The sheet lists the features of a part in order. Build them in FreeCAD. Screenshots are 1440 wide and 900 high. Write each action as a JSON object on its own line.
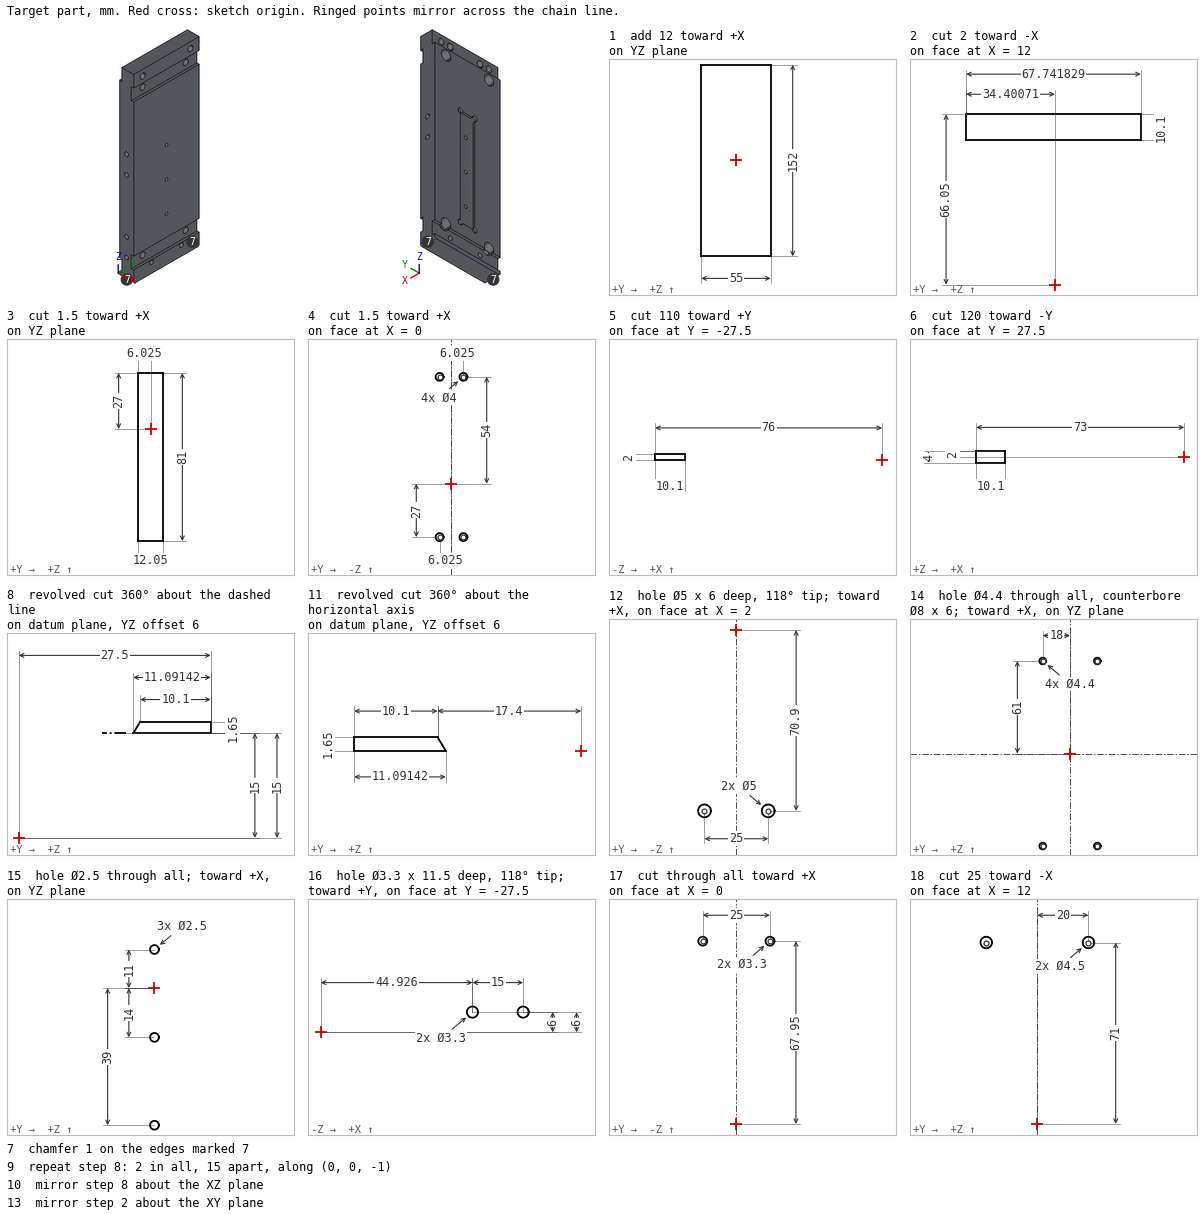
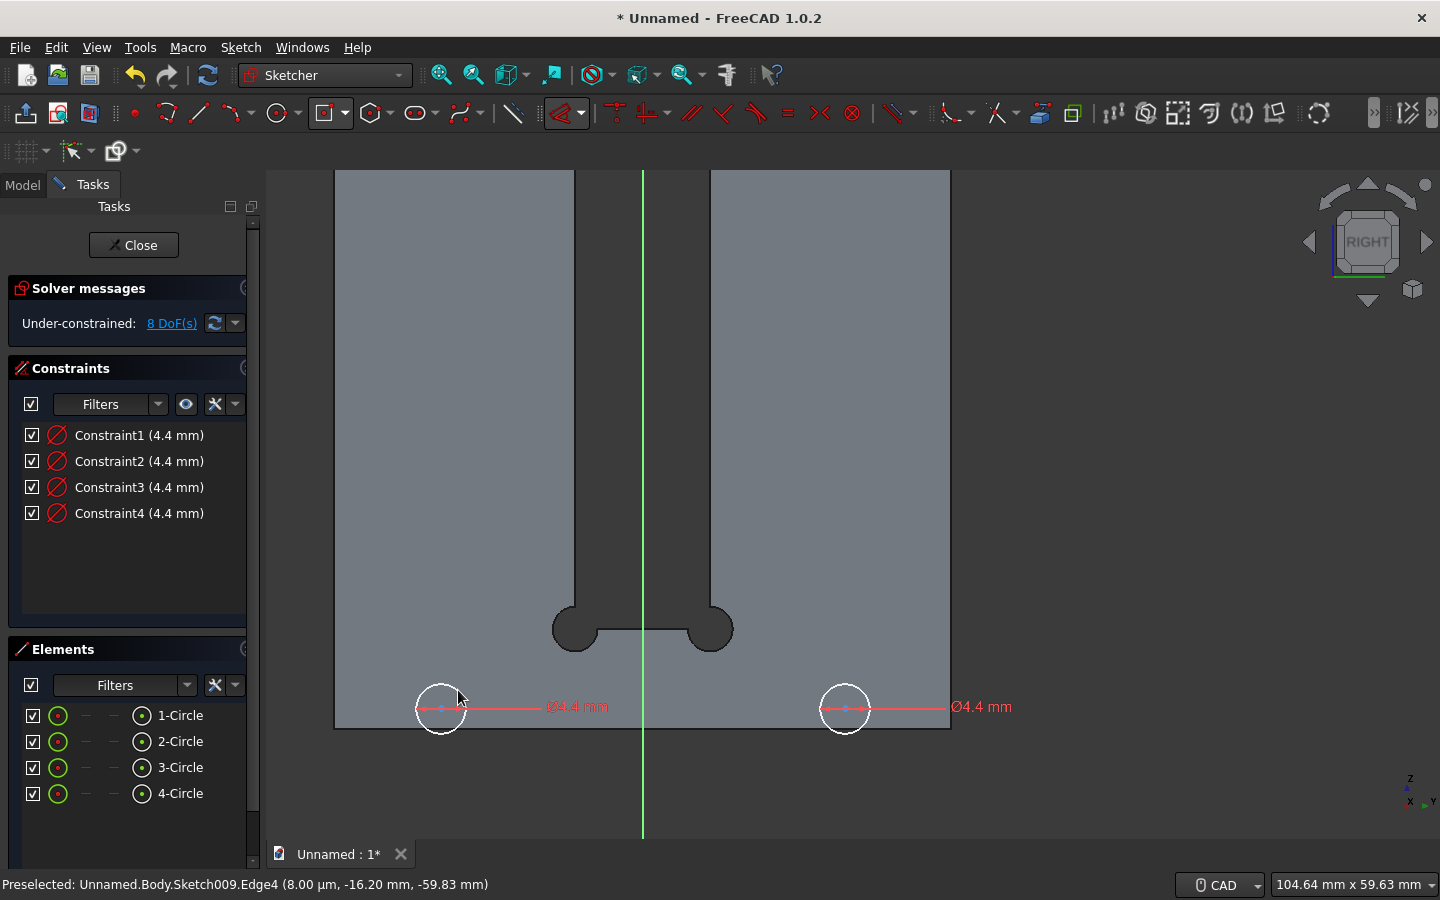
{"action": "scroll", "coordinate": [846, 712], "scroll_direction": "down", "scroll_amount": 6}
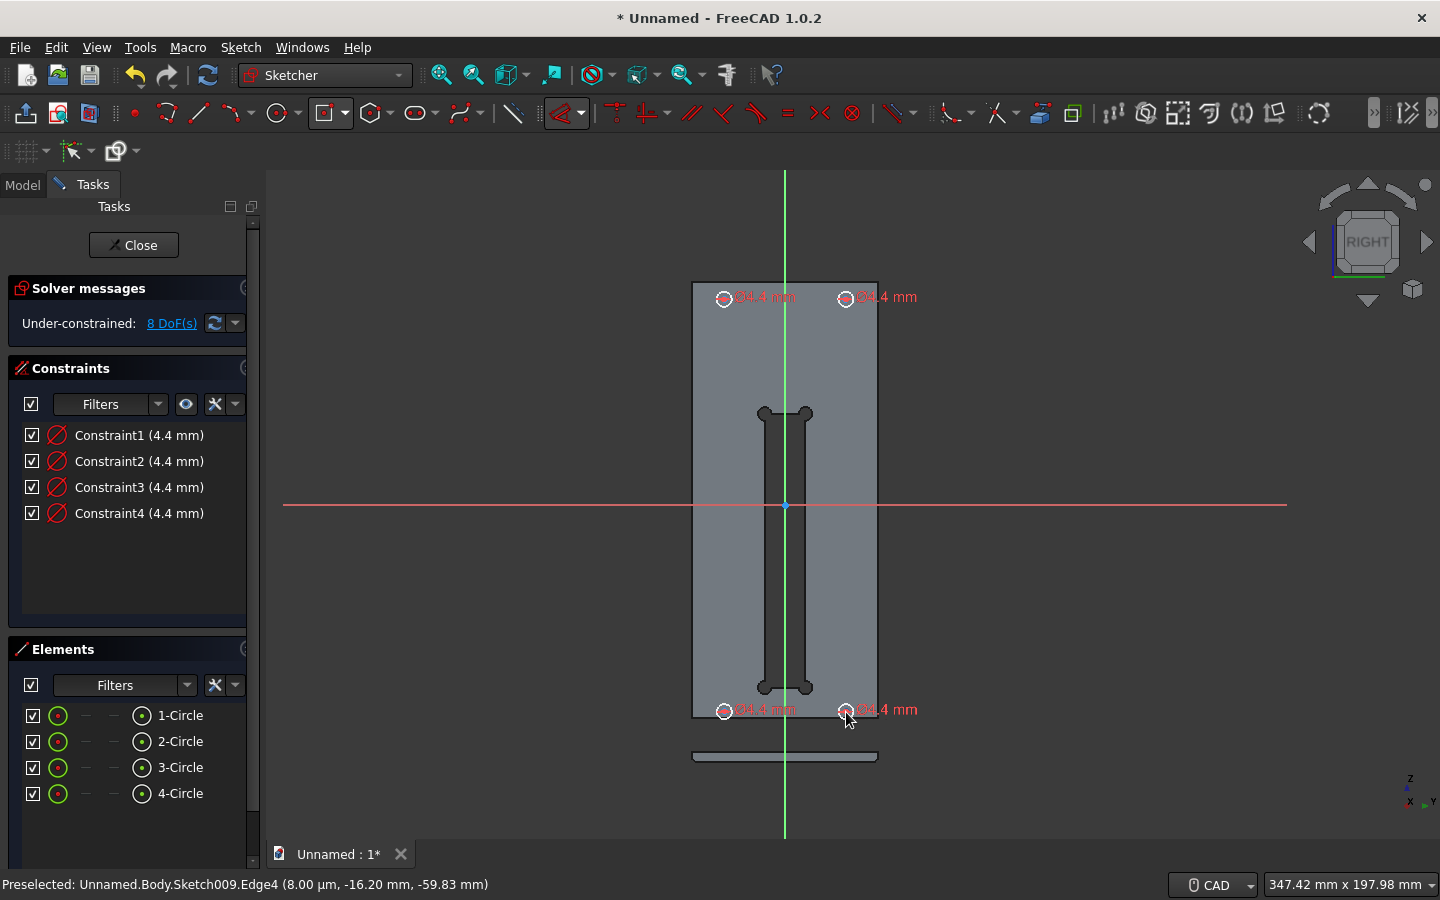
{"action": "left_click", "coordinate": [724, 299]}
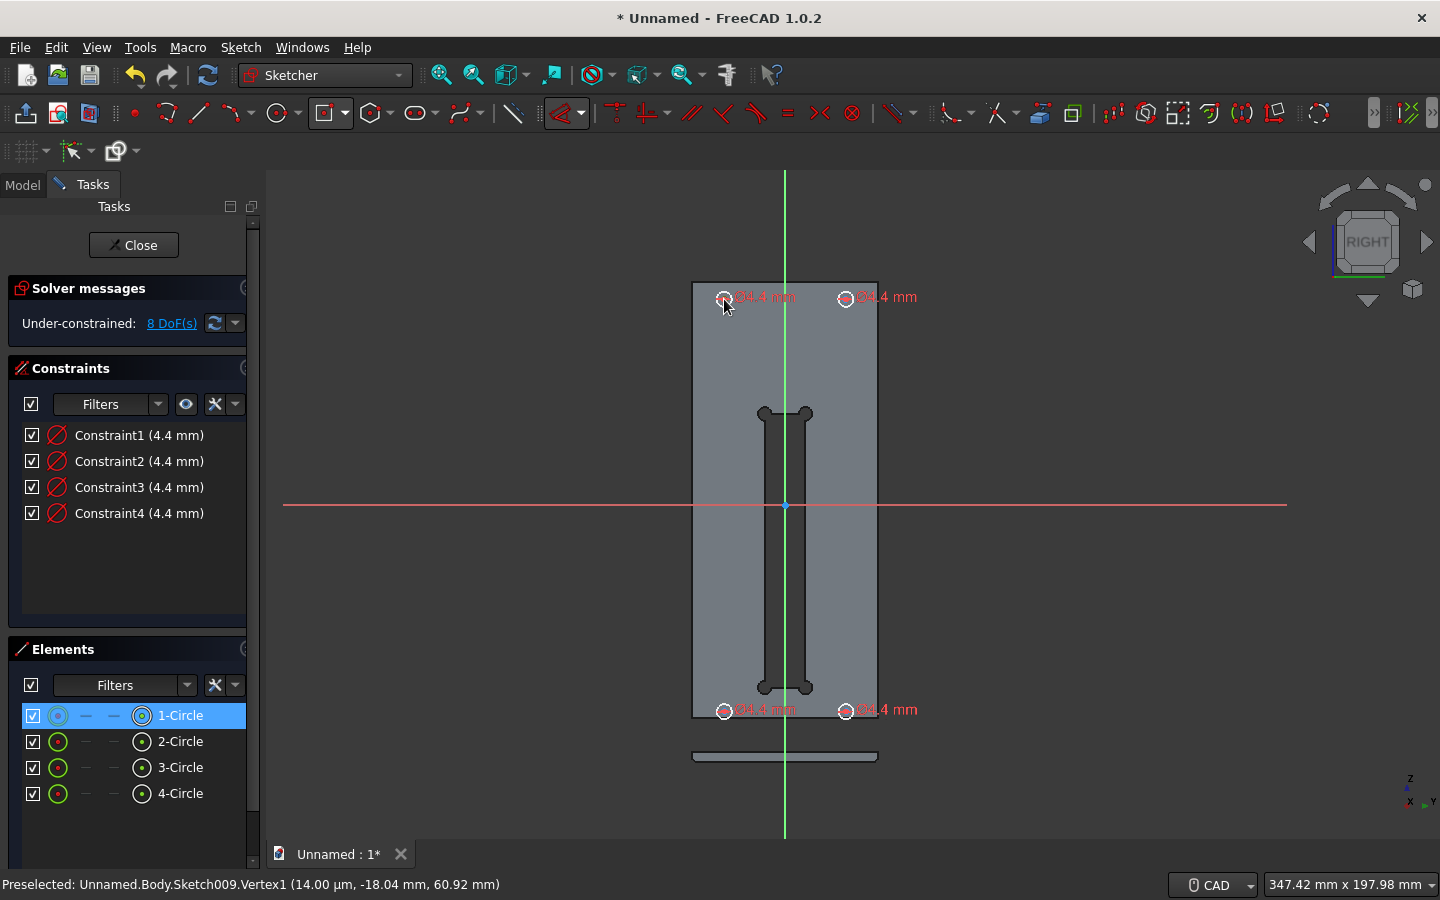
{"action": "left_click", "coordinate": [846, 299]}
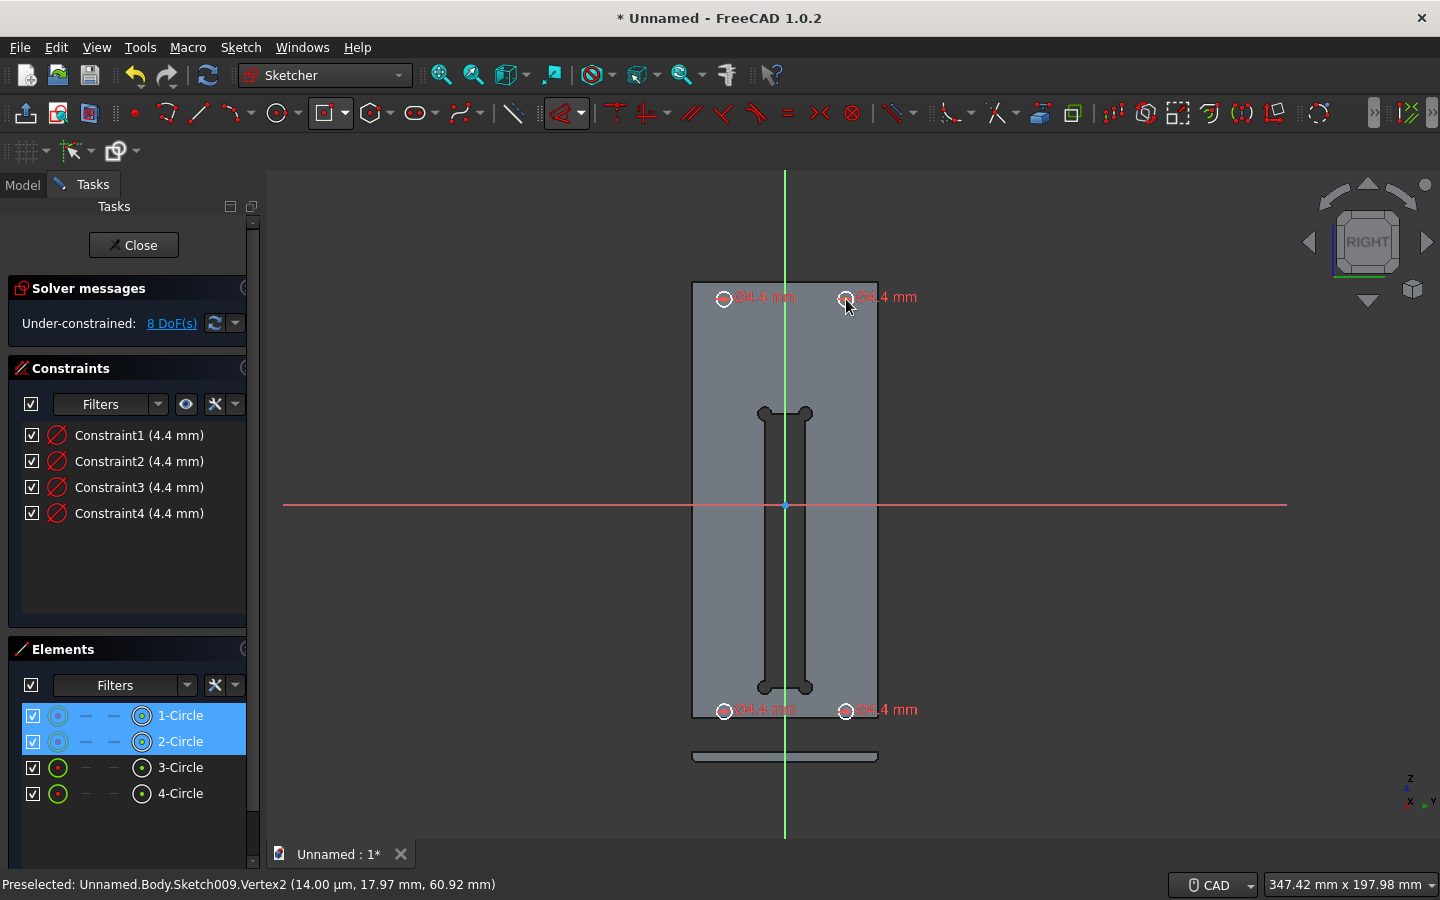
{"action": "left_click", "coordinate": [785, 767]}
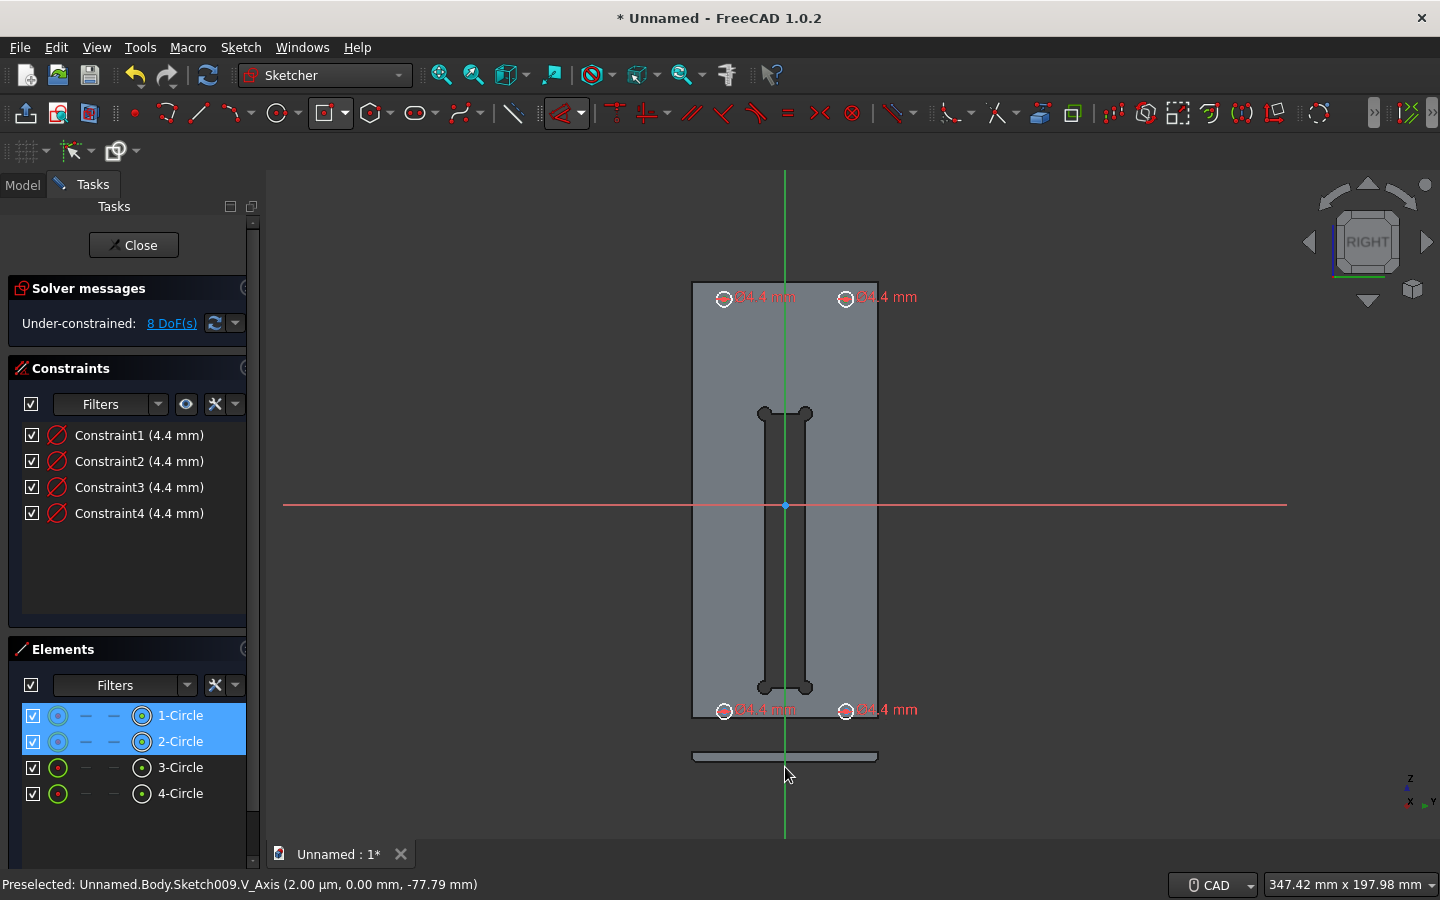
{"action": "left_click", "coordinate": [820, 114]}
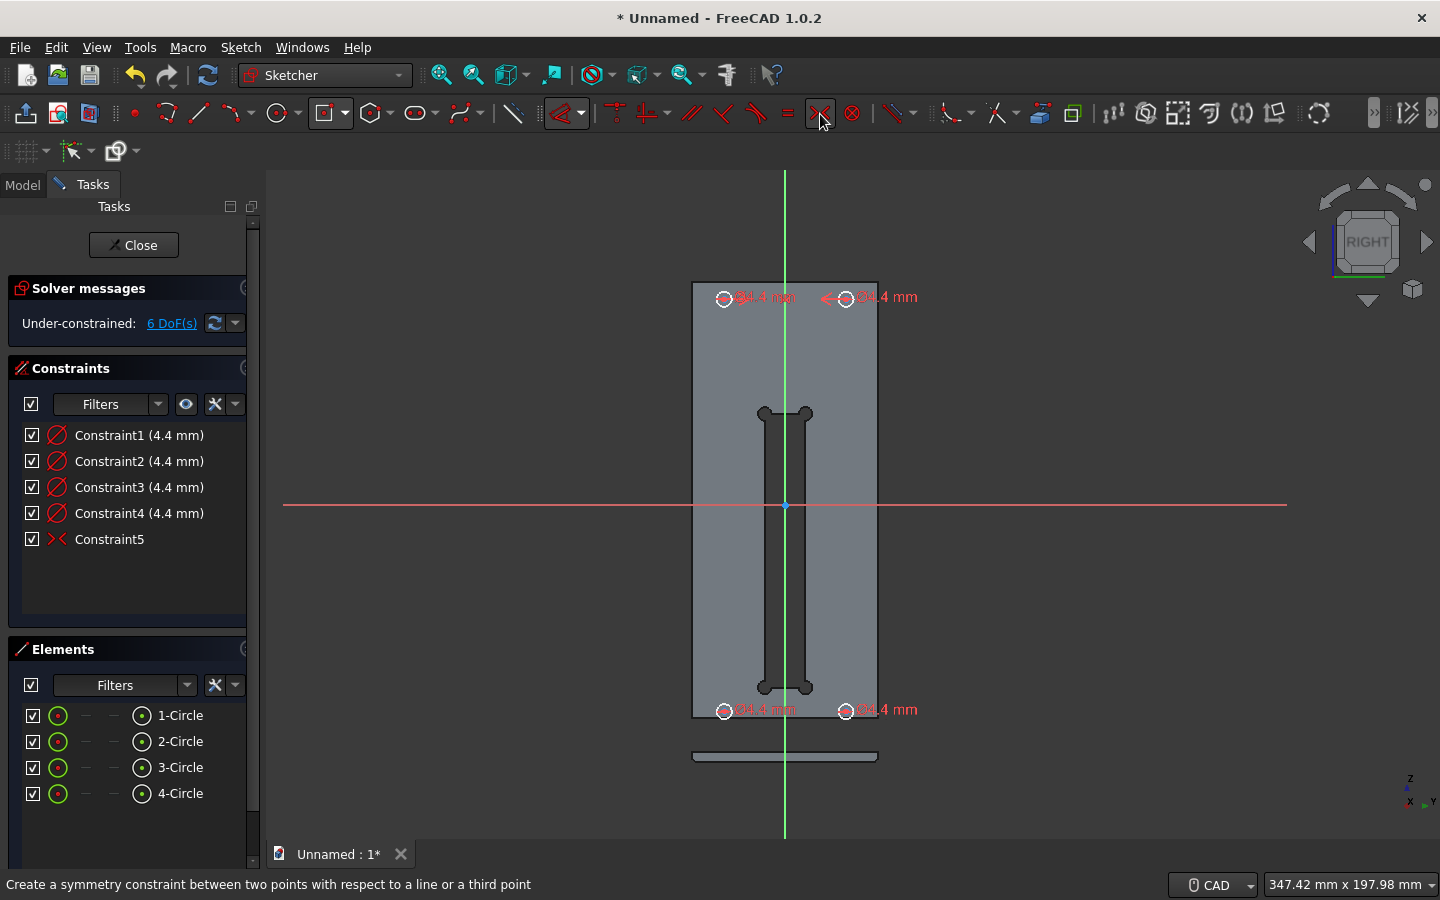
{"action": "left_click", "coordinate": [846, 299]}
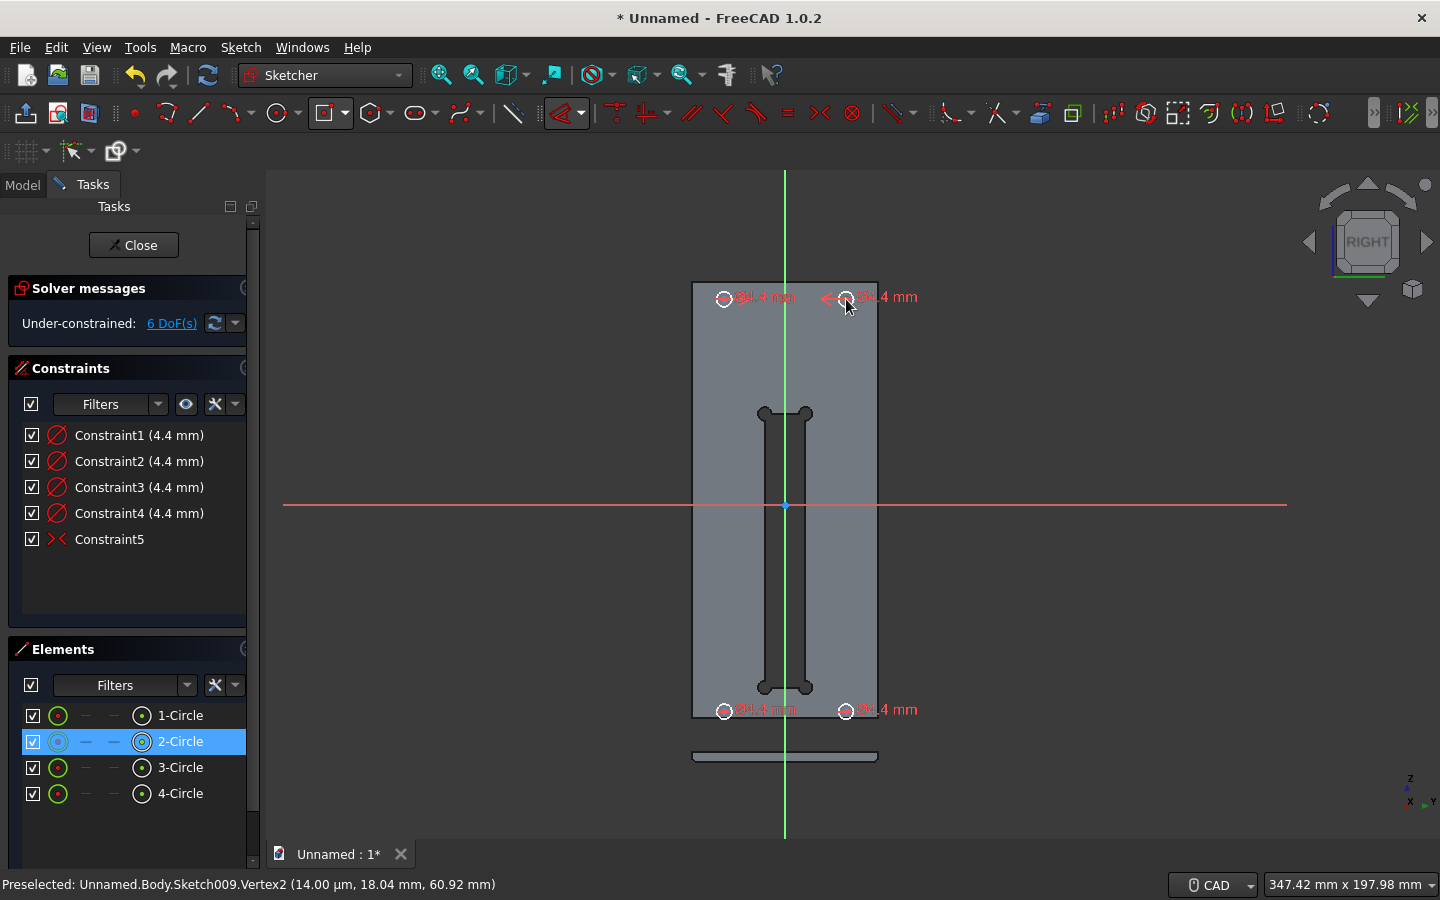
{"action": "left_click", "coordinate": [846, 712]}